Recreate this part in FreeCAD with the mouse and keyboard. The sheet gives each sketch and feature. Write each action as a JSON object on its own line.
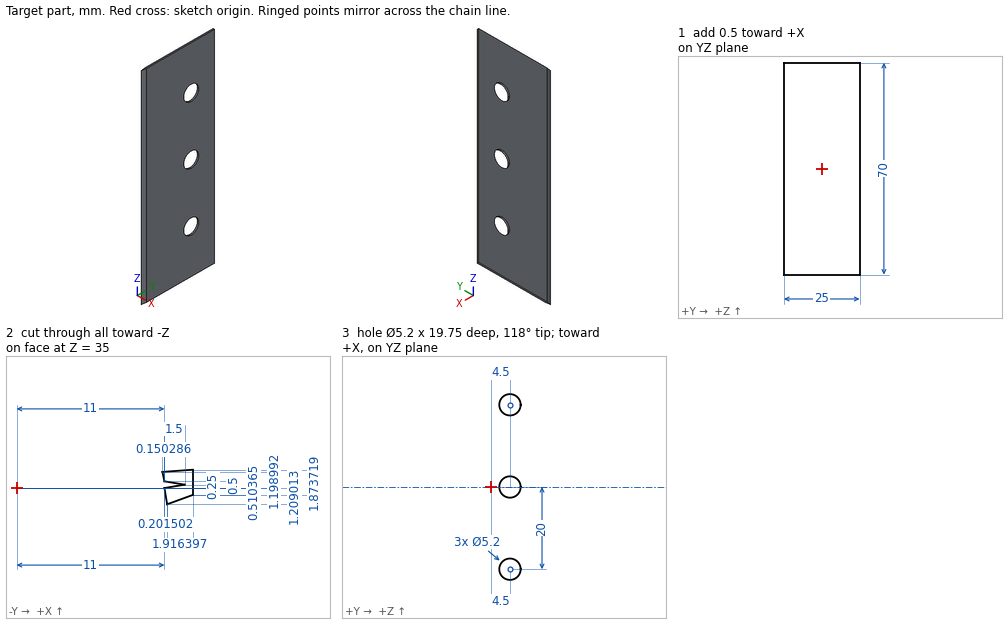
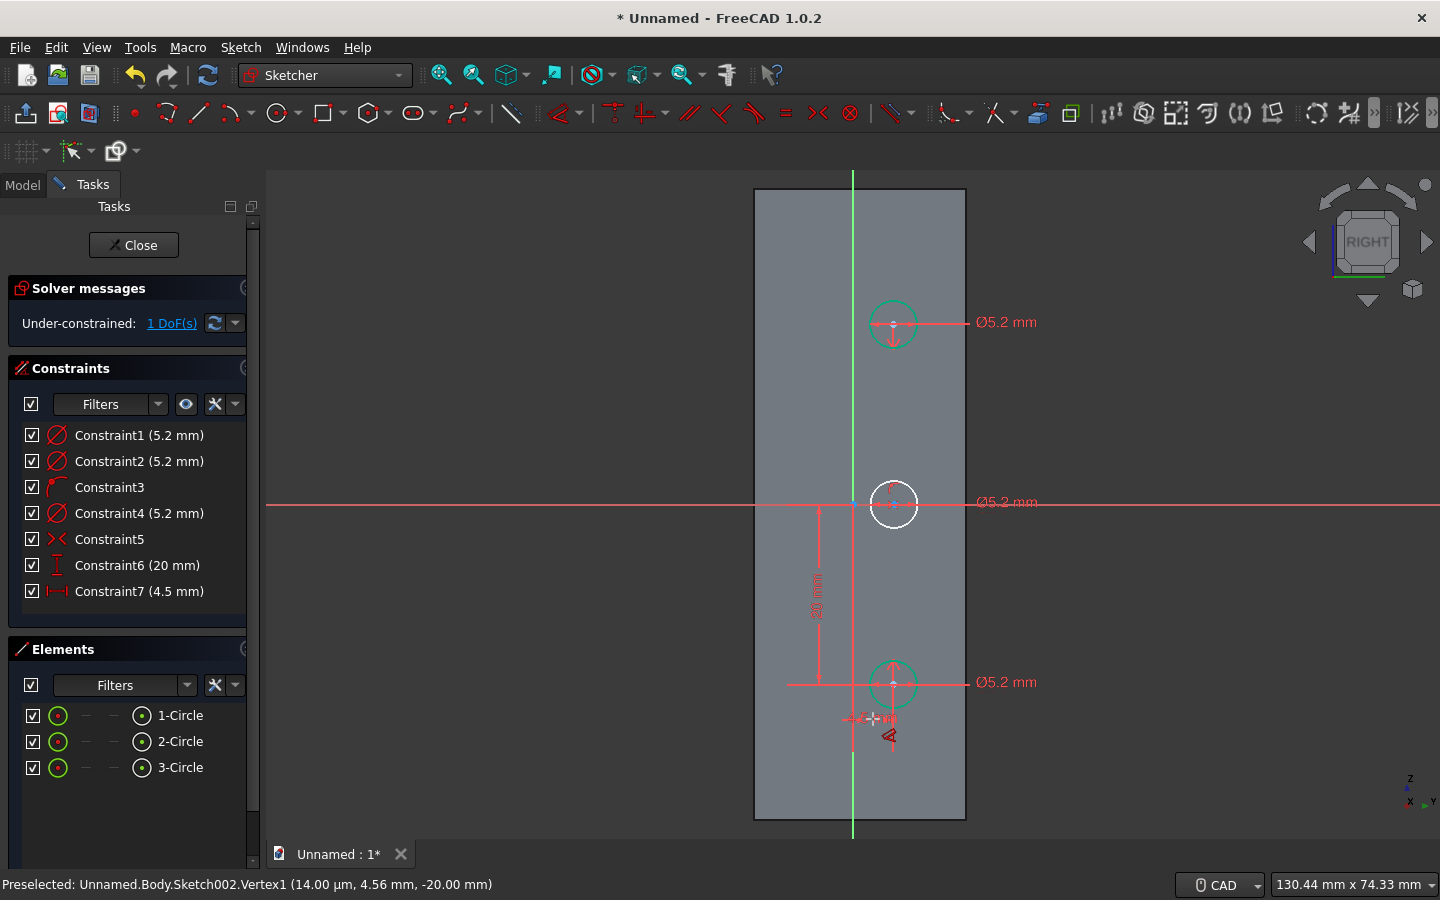
{"action": "left_click", "coordinate": [894, 504]}
{"action": "left_click", "coordinate": [873, 538]}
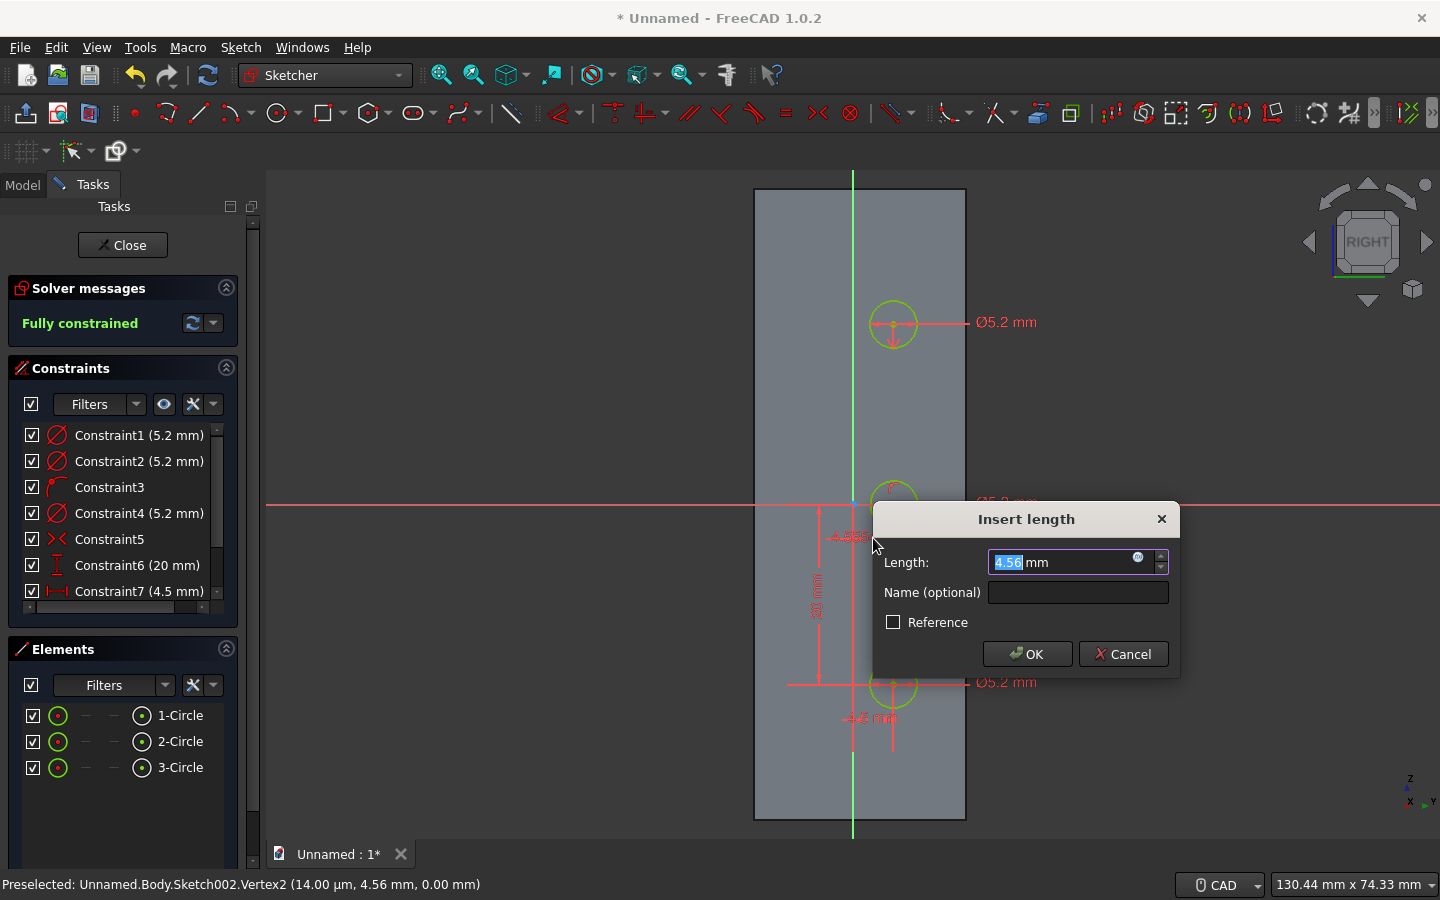
{"action": "type", "text": "4.5"}
{"action": "key", "text": "Return"}
{"action": "key", "text": "Escape"}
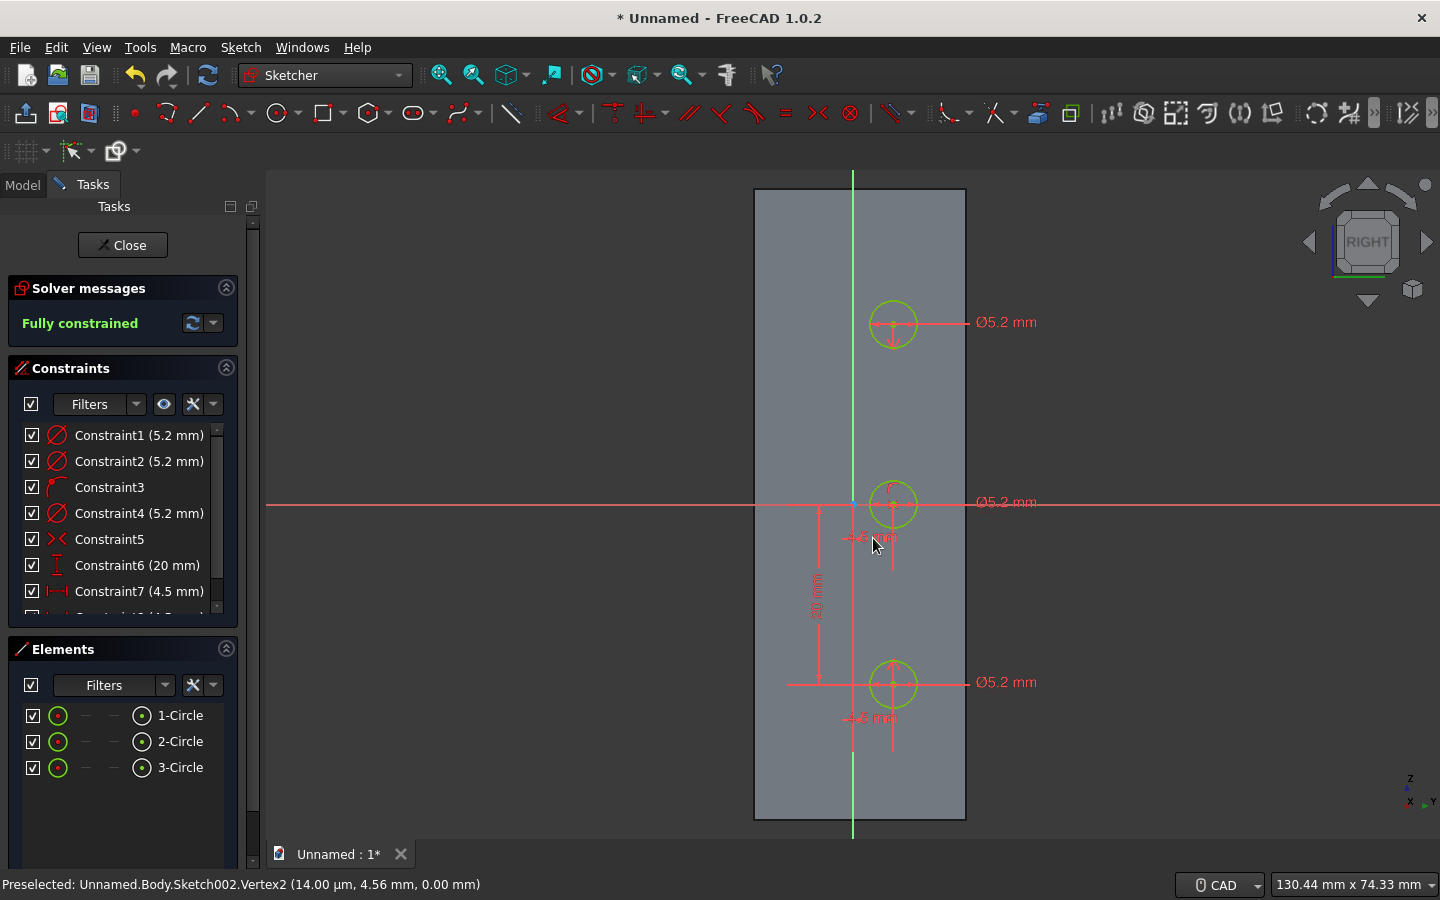
{"action": "left_click", "coordinate": [123, 245]}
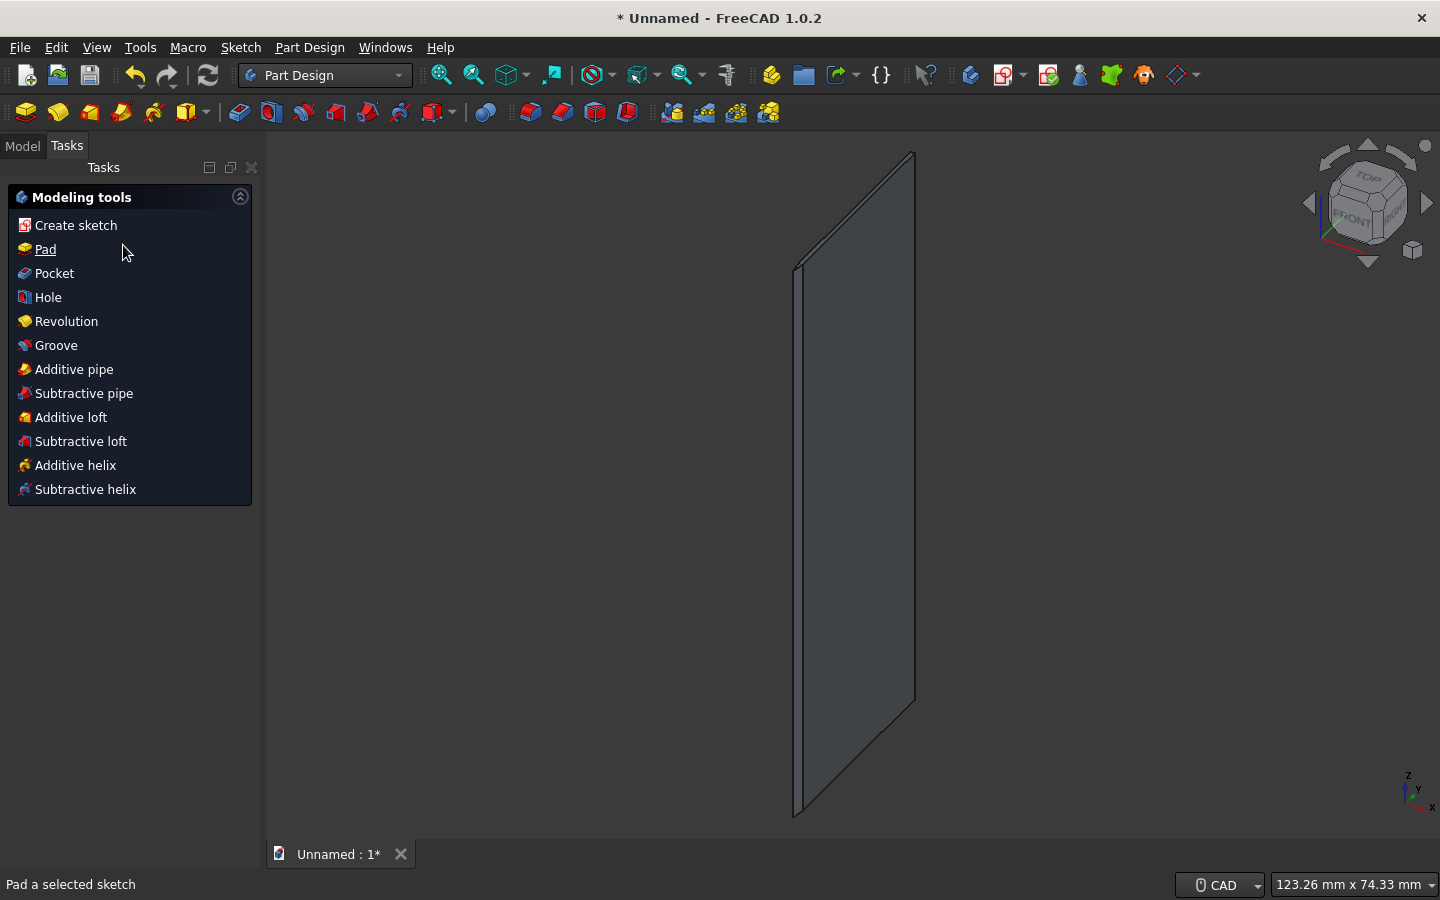
{"action": "left_click", "coordinate": [272, 112]}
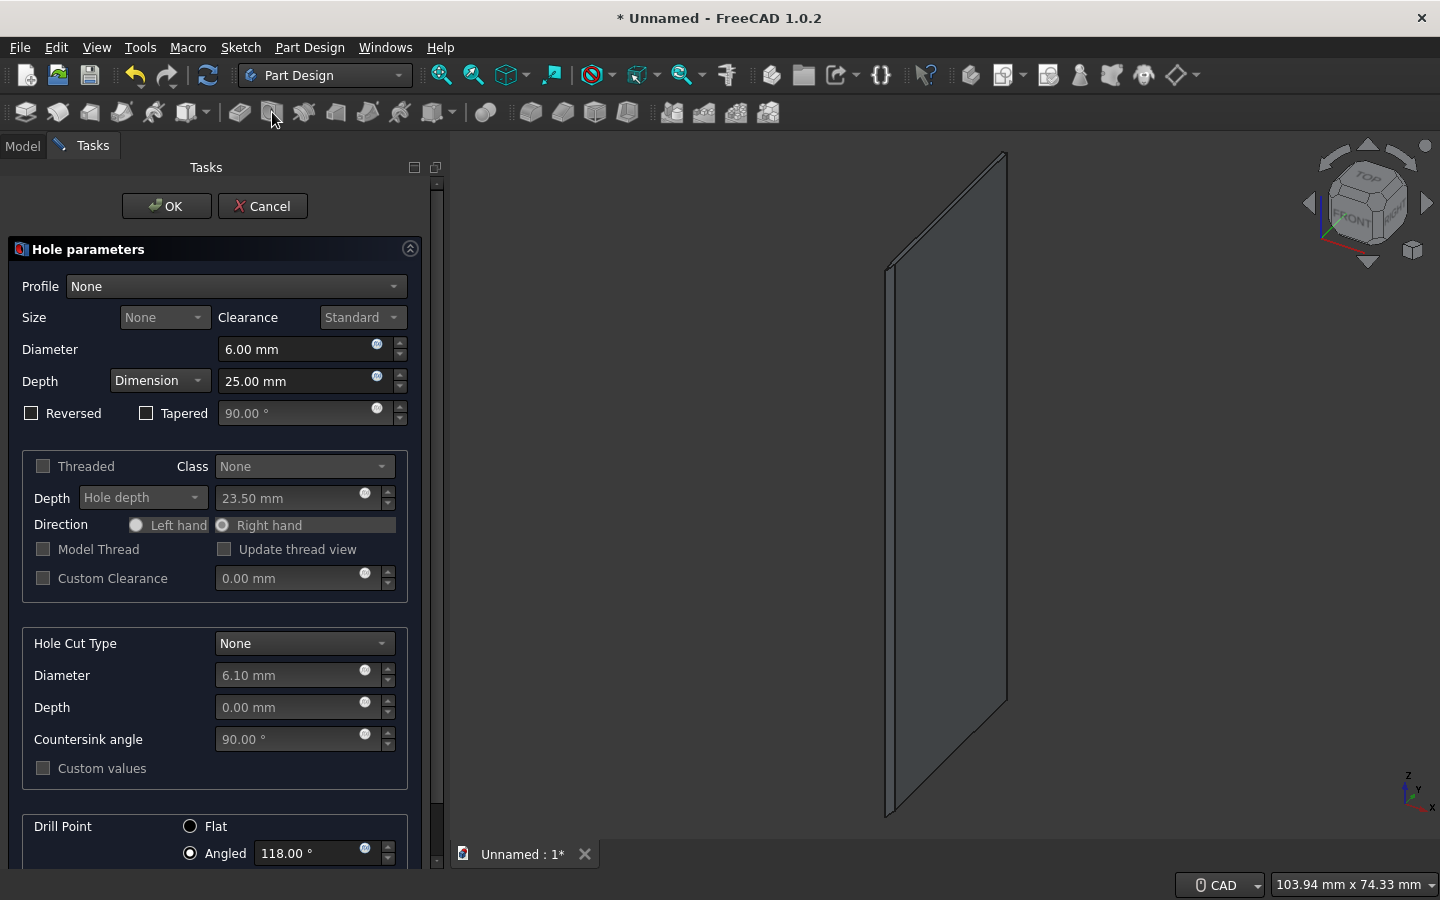
{"action": "triple_click", "coordinate": [305, 349]}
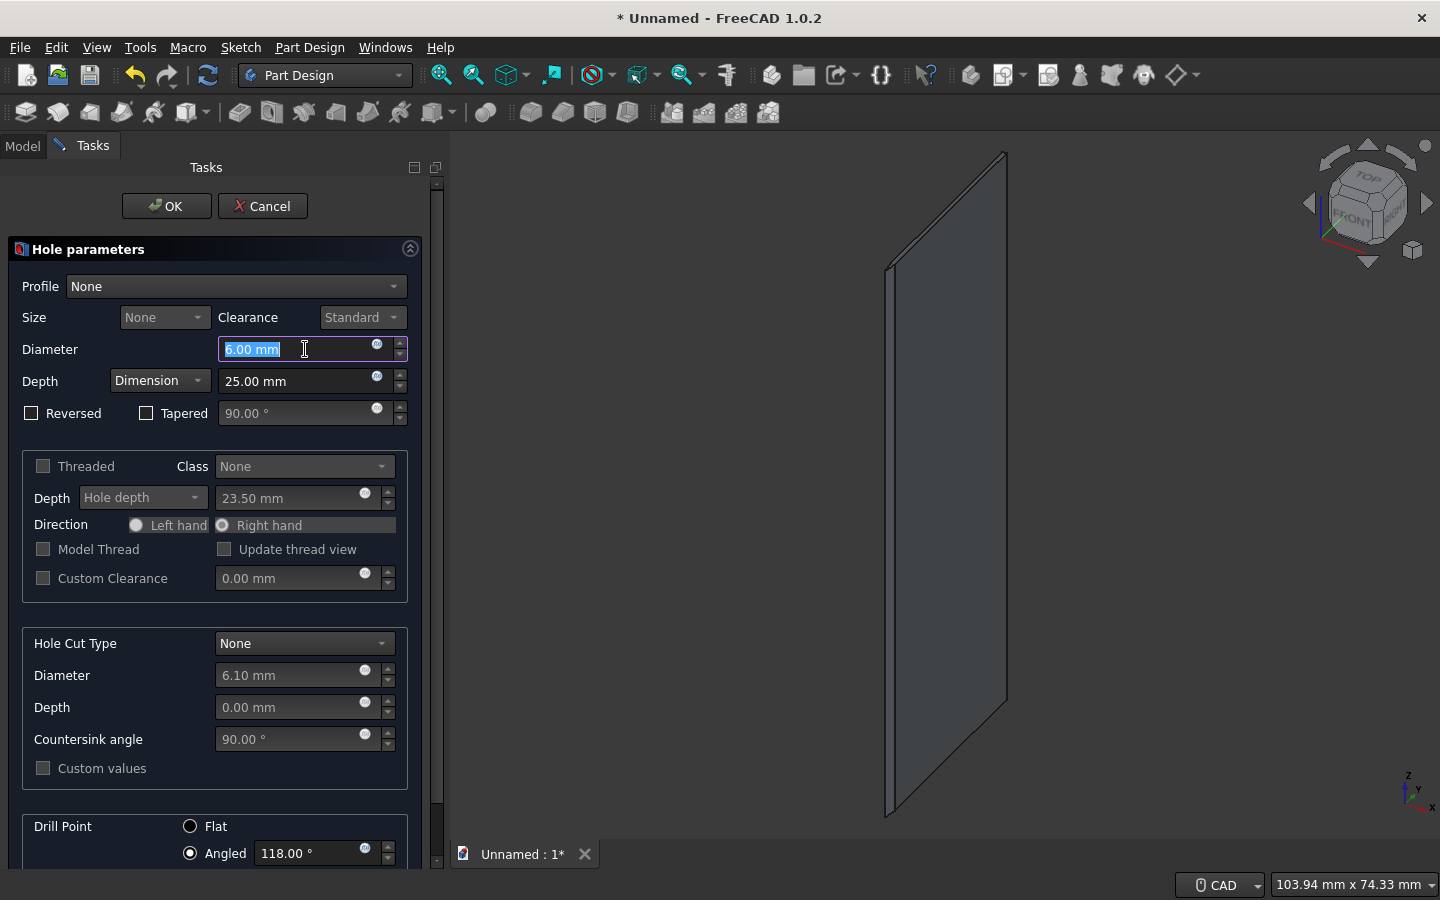
{"action": "type", "text": "5.2"}
{"action": "key", "text": "Tab"}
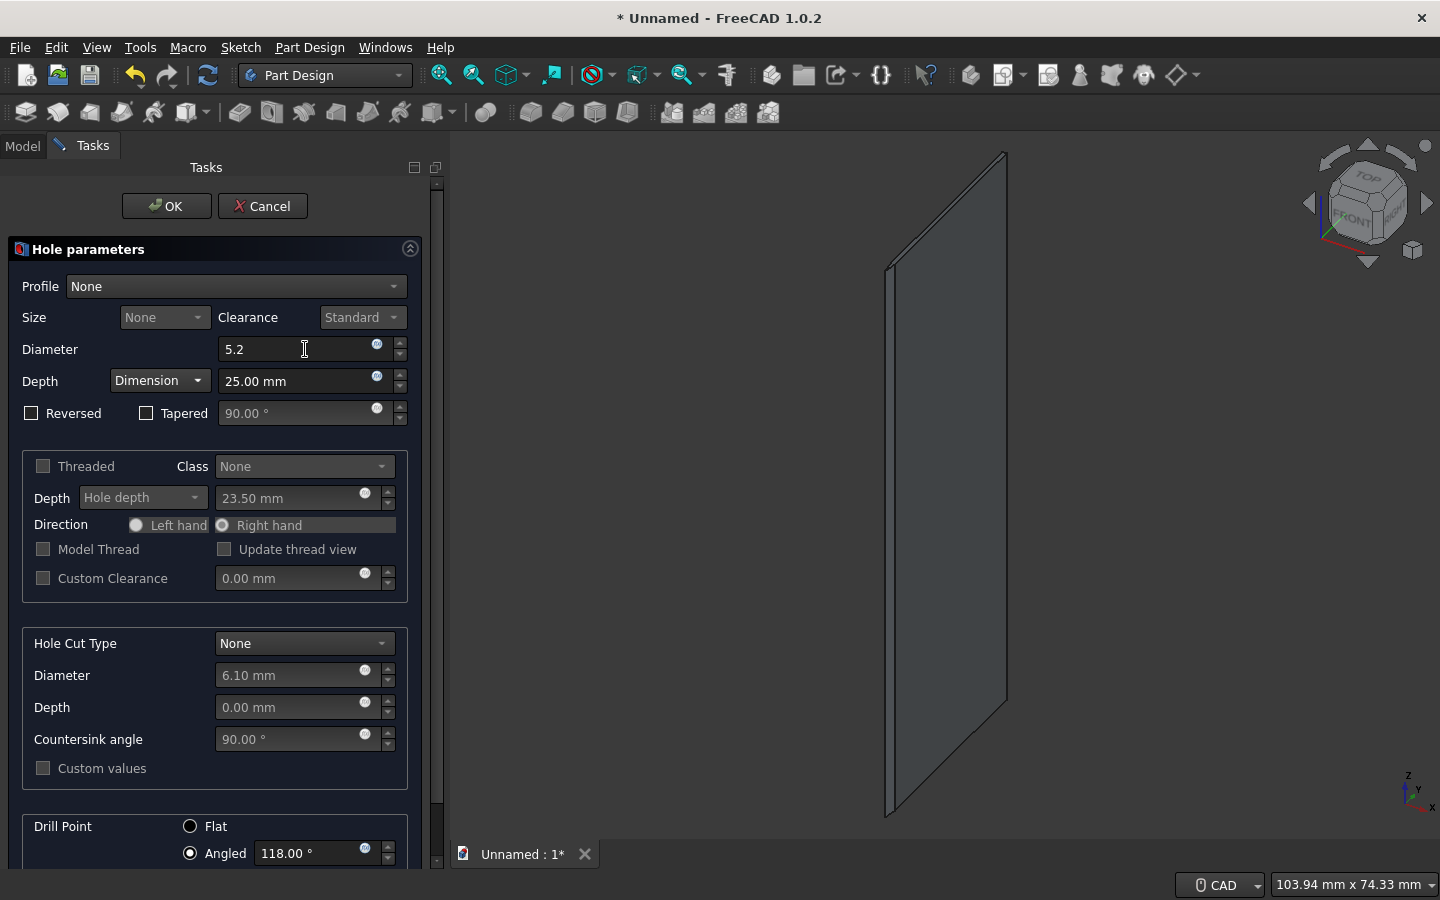
{"action": "triple_click", "coordinate": [305, 381]}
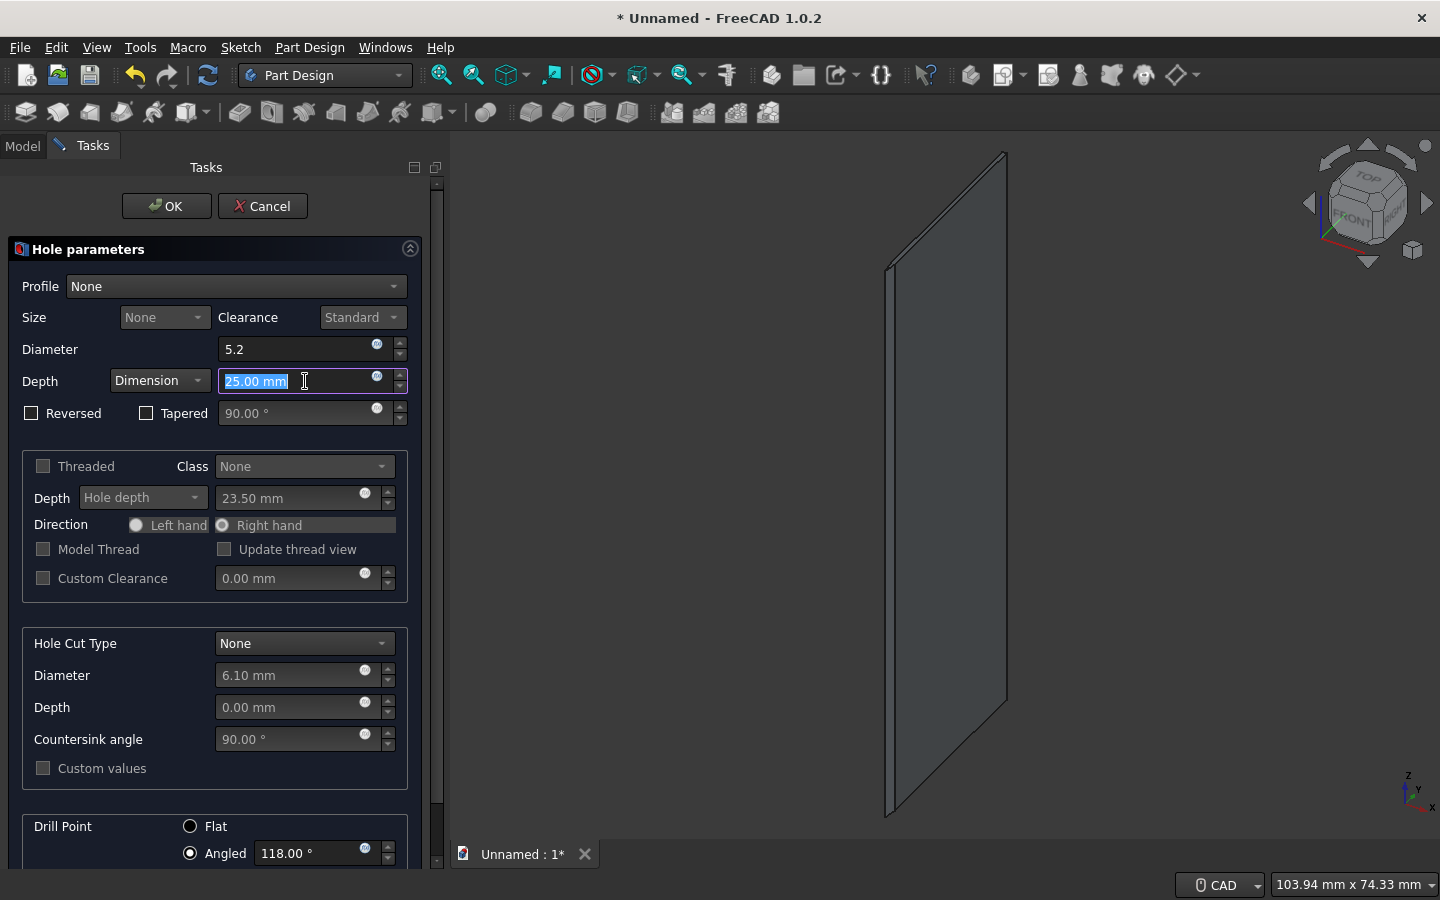
{"action": "type", "text": "19.75"}
{"action": "key", "text": "Tab"}